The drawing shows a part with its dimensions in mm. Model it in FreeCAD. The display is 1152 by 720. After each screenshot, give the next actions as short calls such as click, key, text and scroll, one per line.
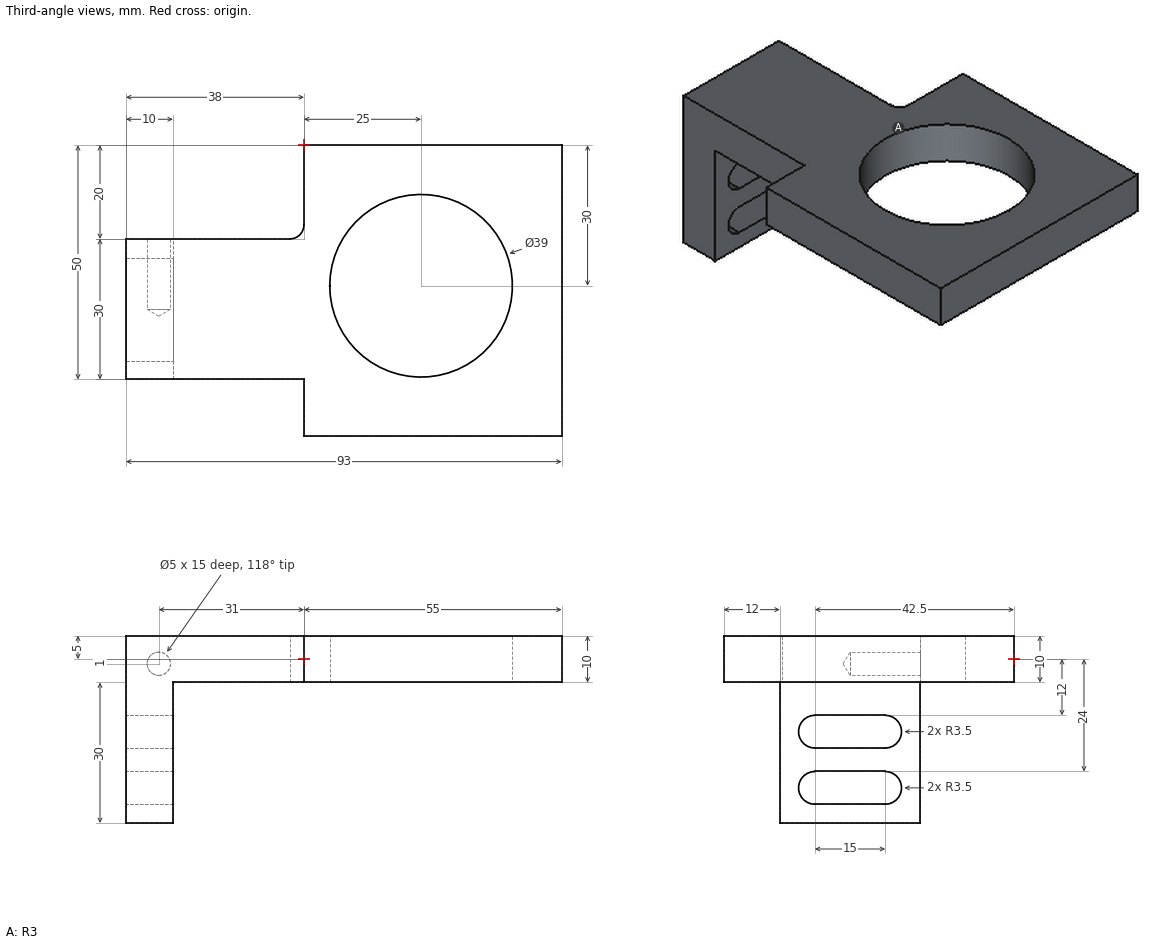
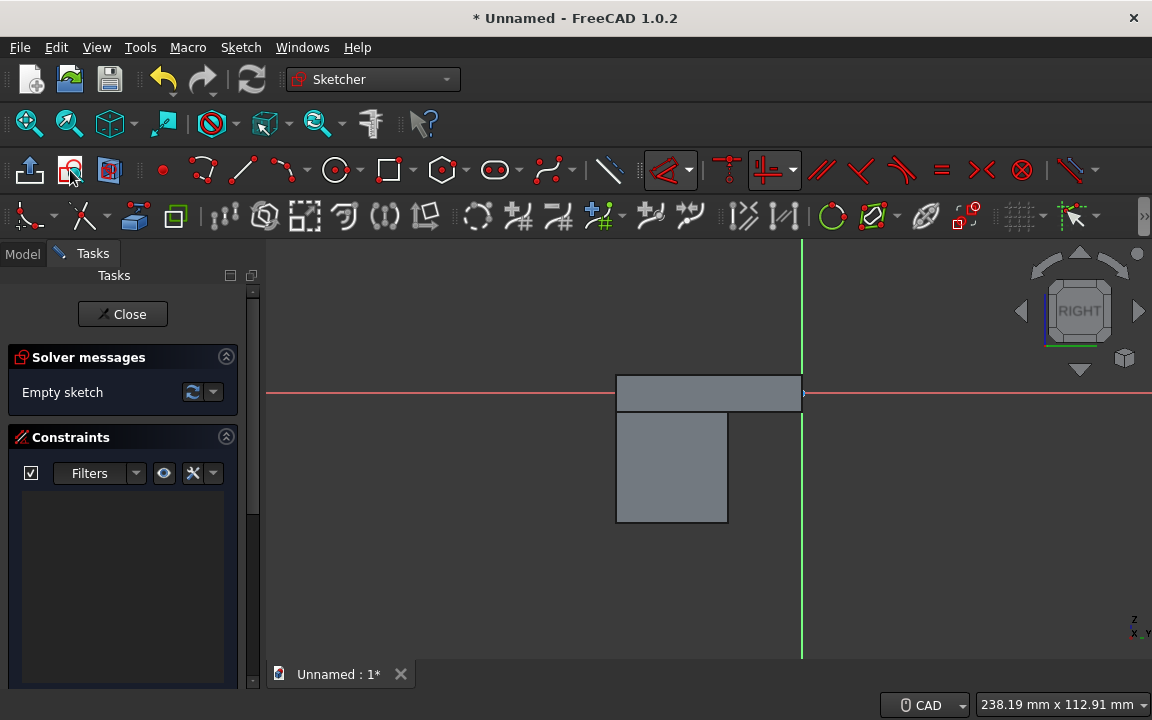
click(110, 170)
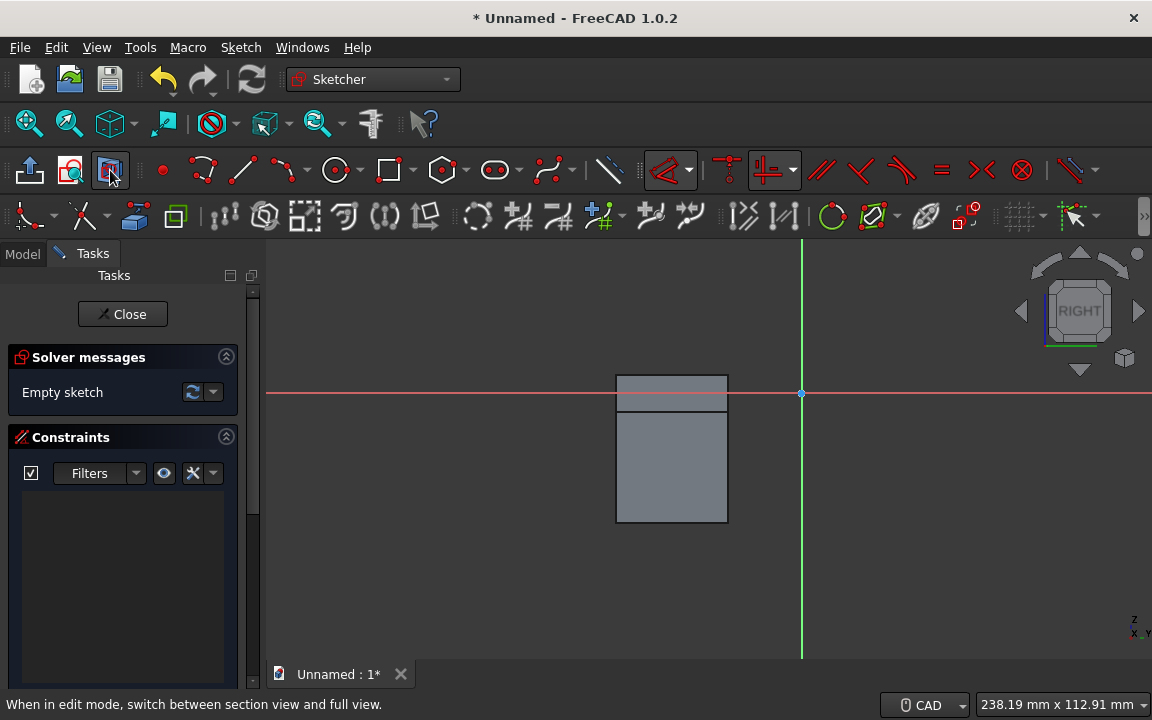
scroll(778, 452, up, 4)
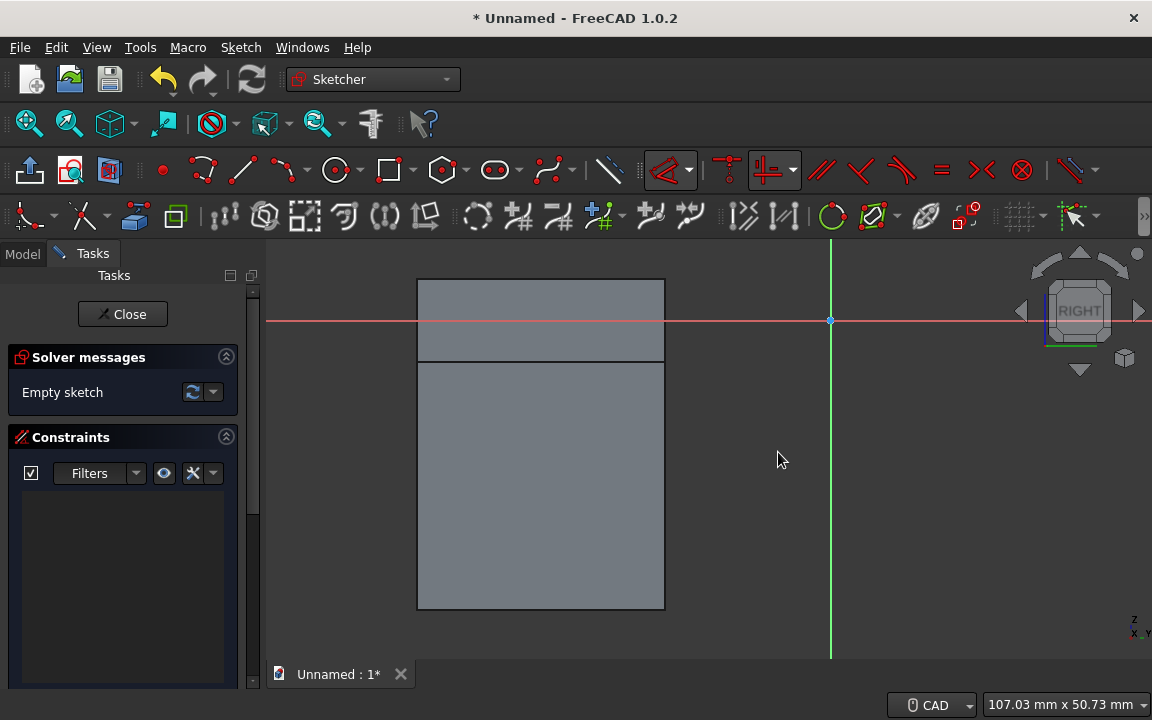
key(g)
key(s)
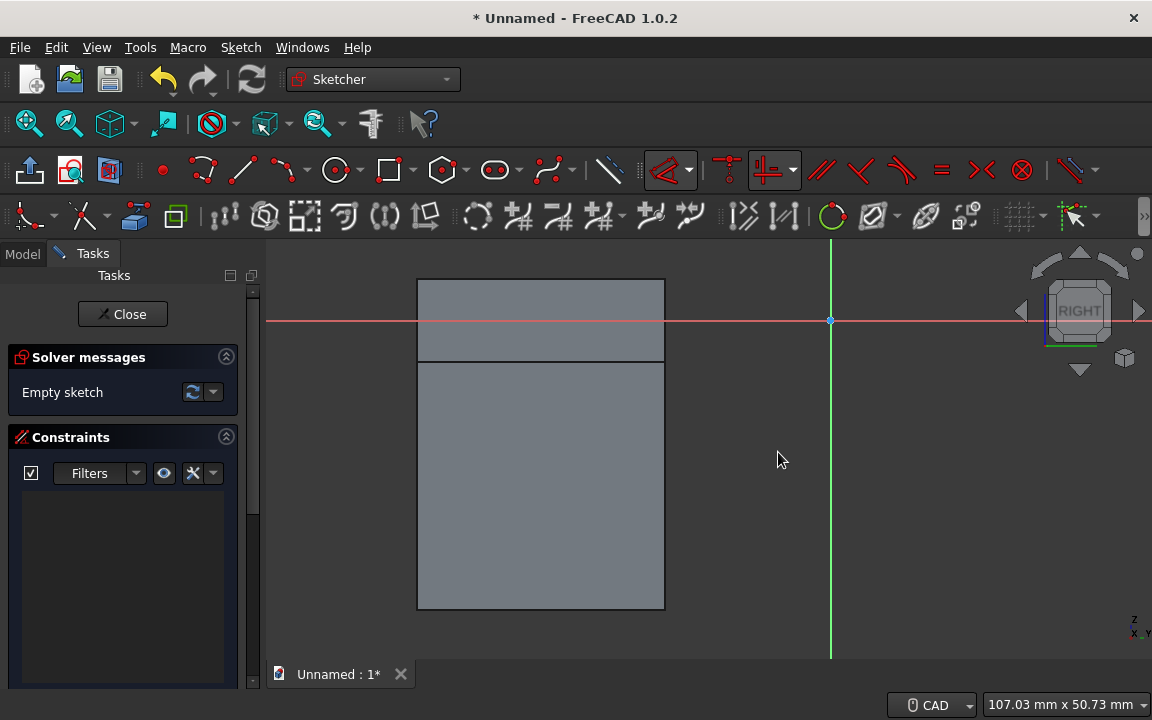
click(479, 548)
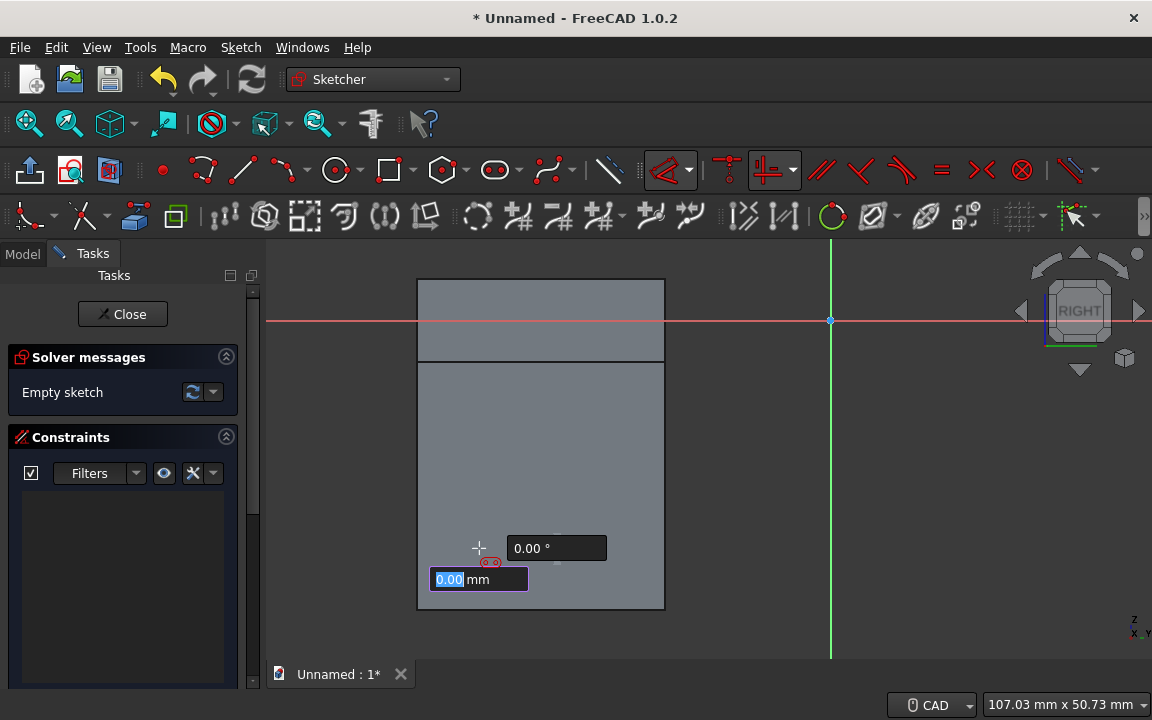
click(603, 548)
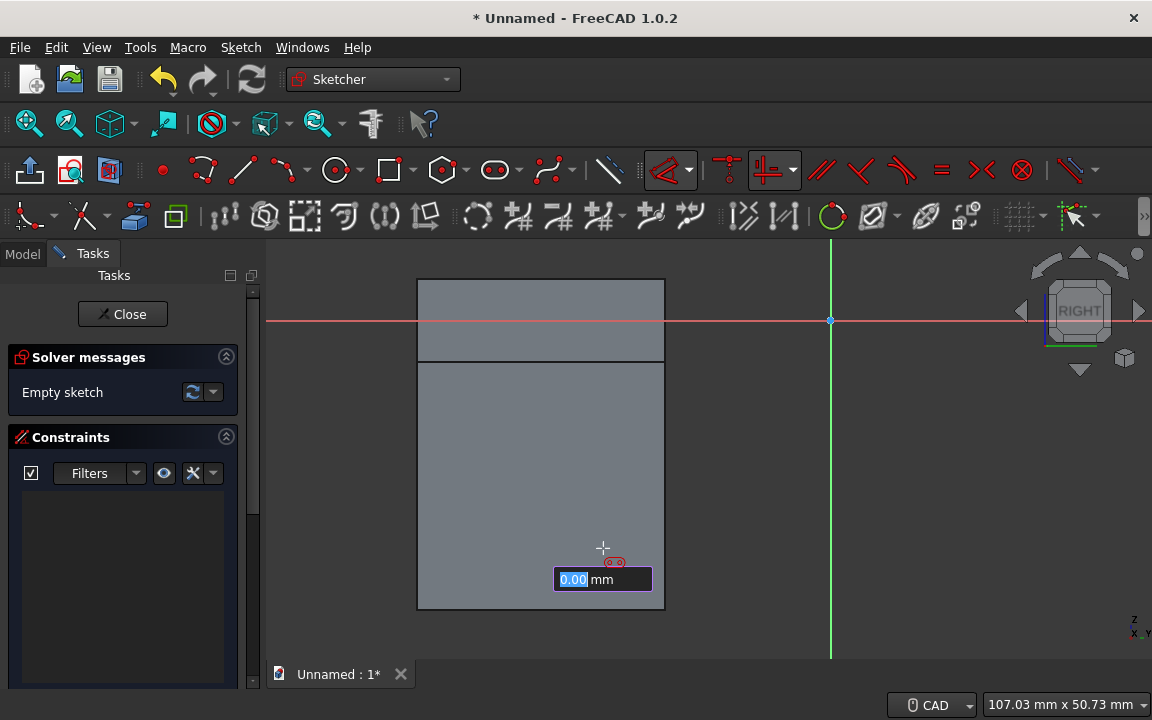
click(541, 577)
key(Escape)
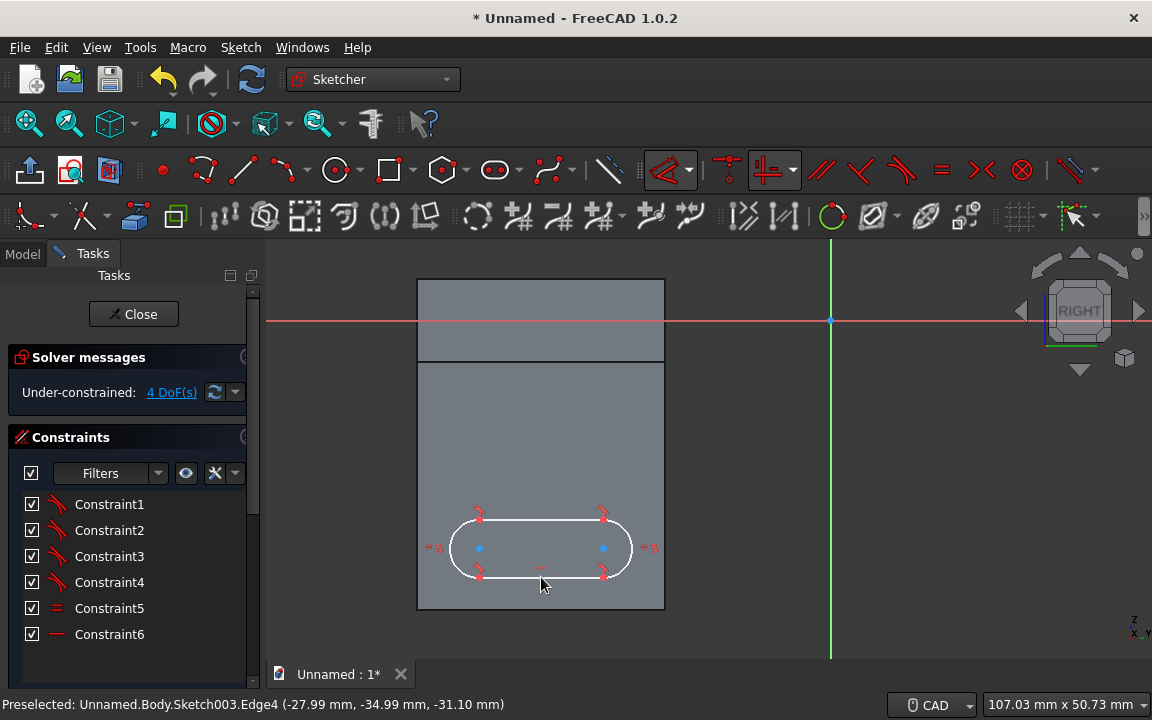
scroll(456, 532, up, 2)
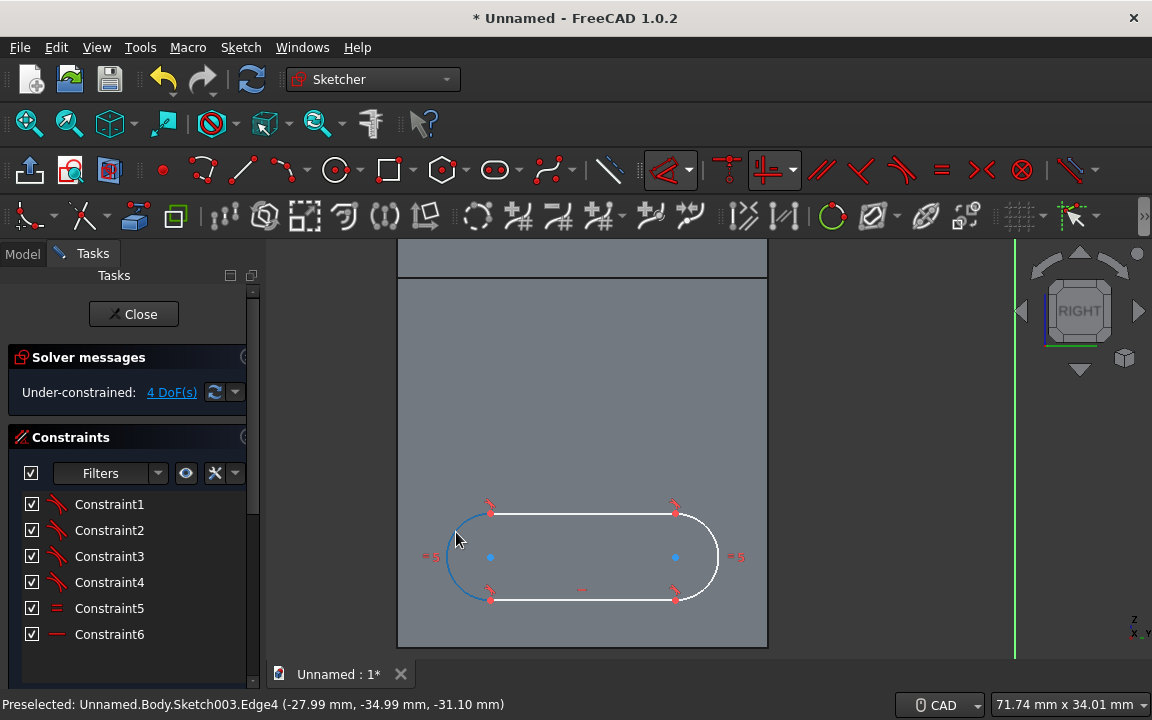
click(455, 532)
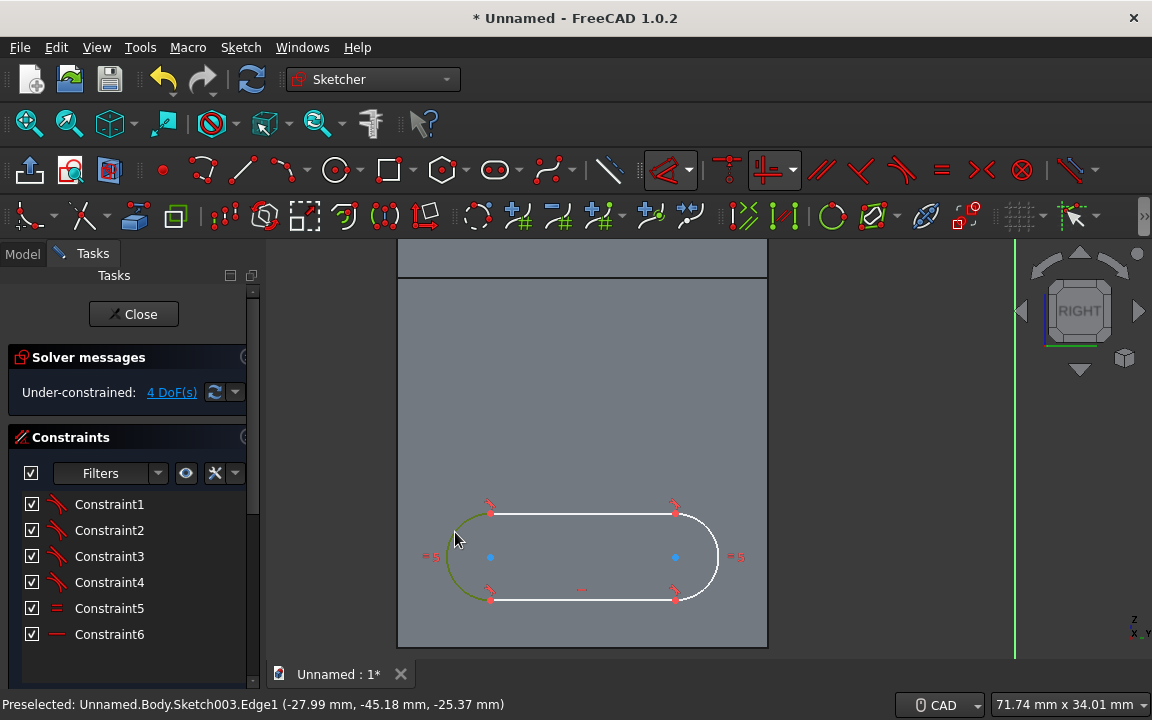
key(k)
key(r)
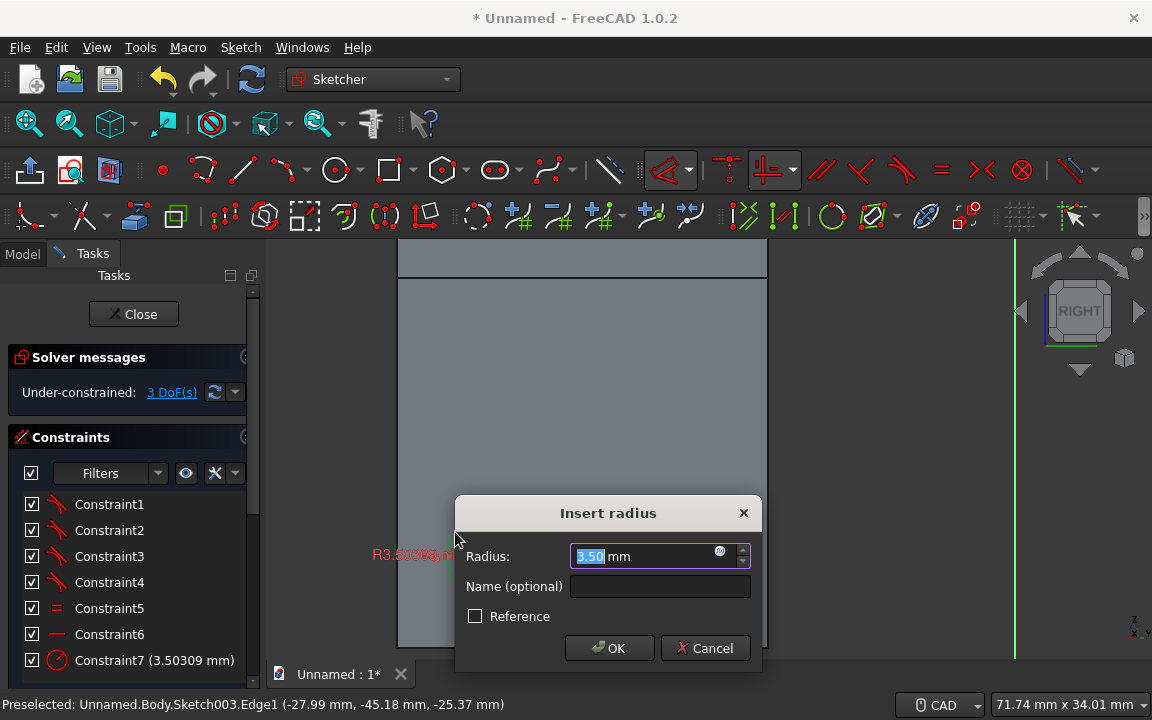
text(3.5)
key(Return)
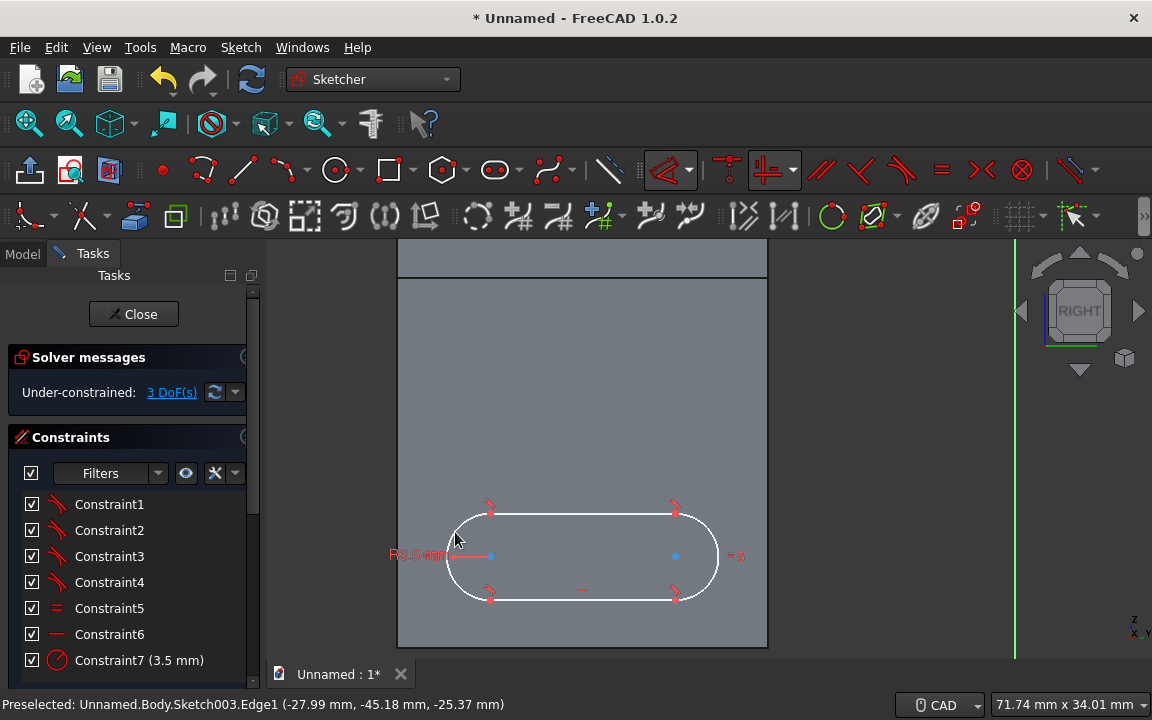
click(546, 514)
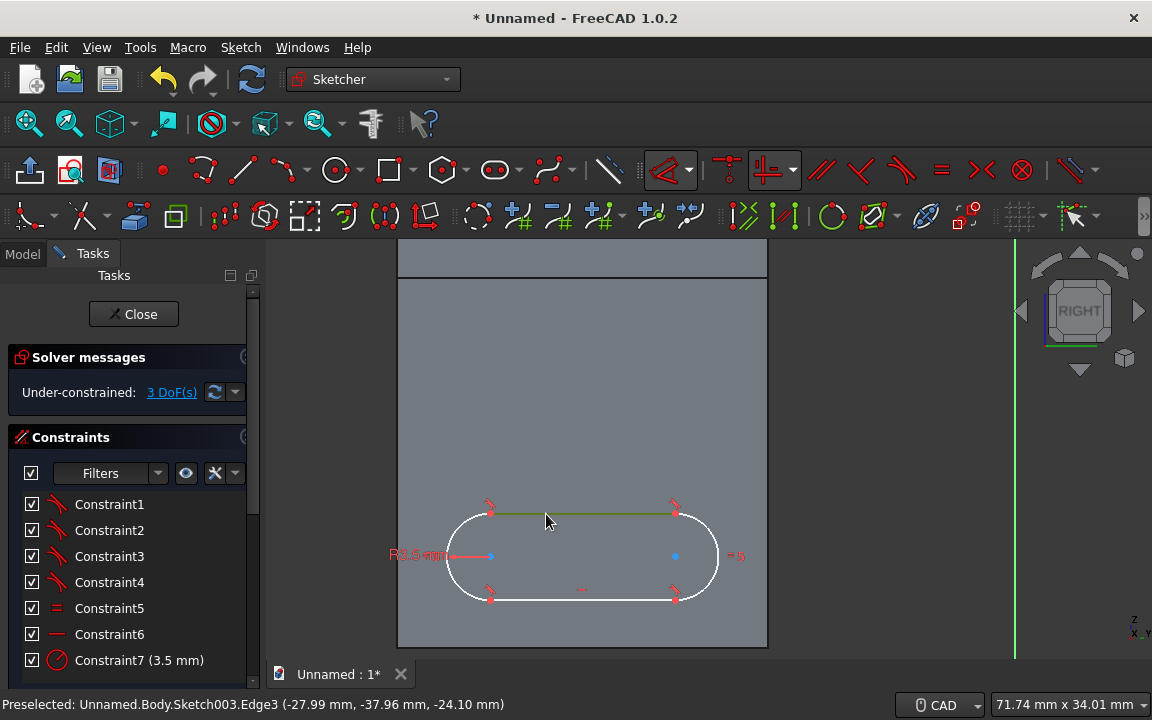
key(l)